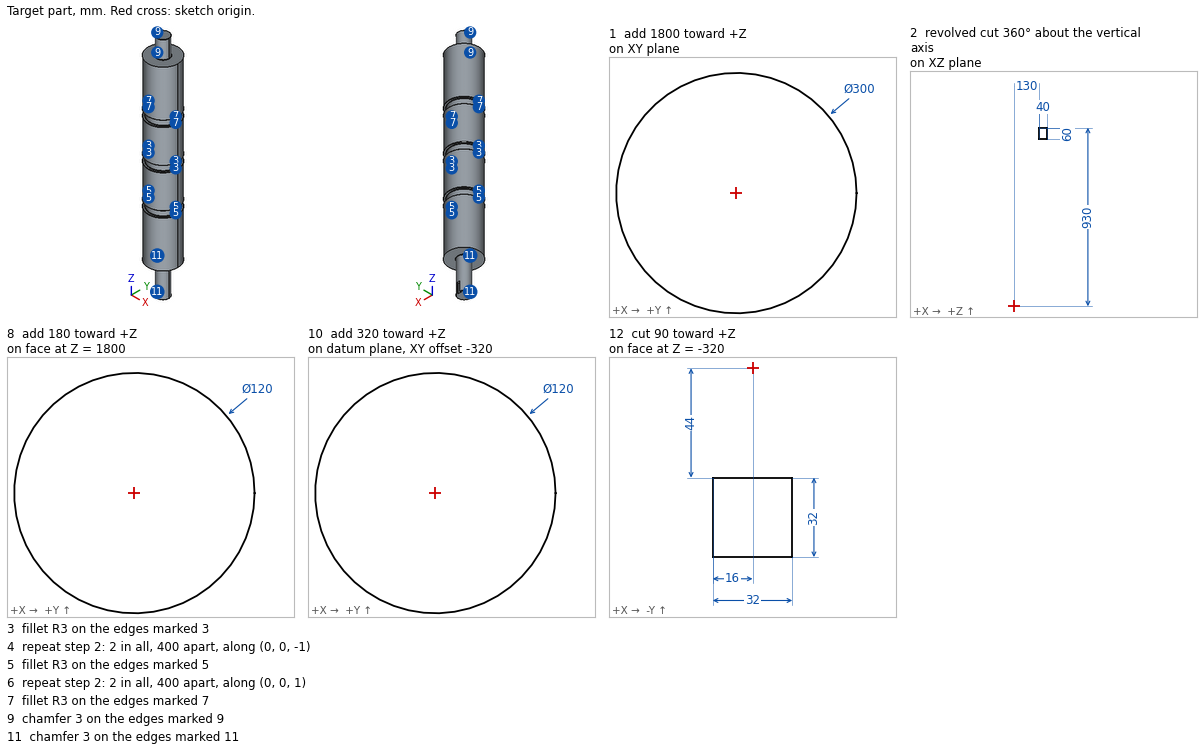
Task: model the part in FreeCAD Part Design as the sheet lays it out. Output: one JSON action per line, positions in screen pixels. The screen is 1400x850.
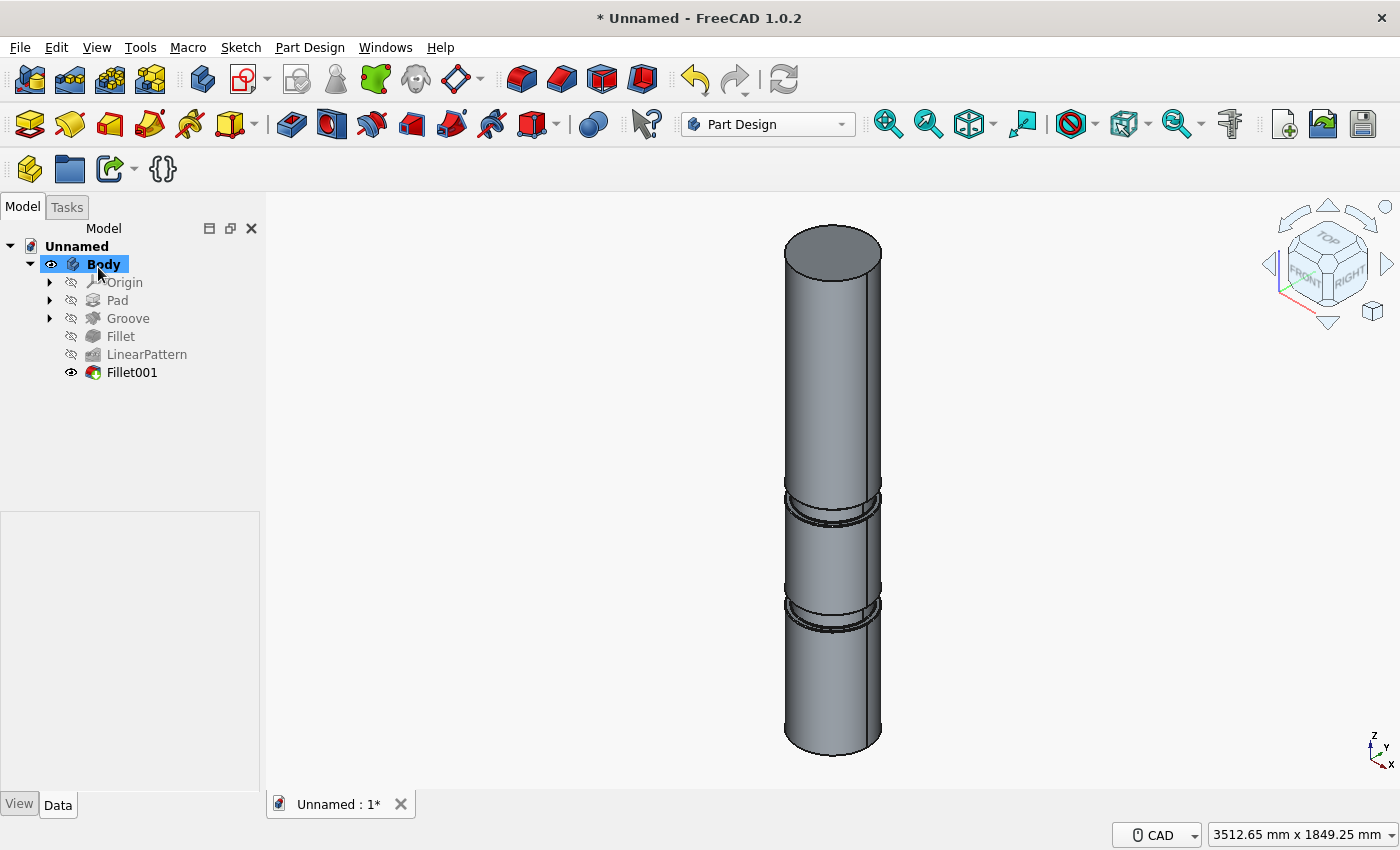
{"action": "left_click", "coordinate": [116, 318]}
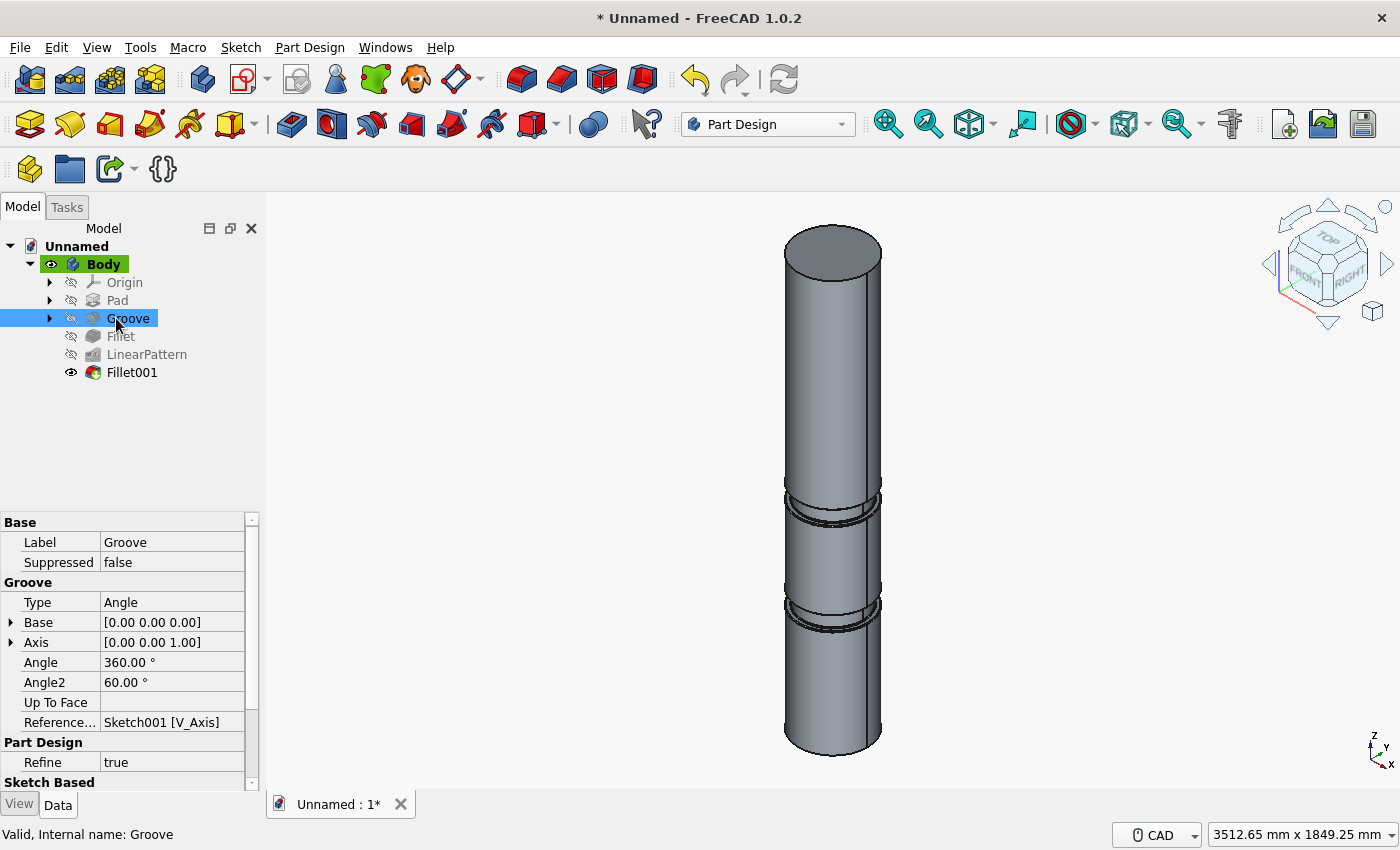
{"action": "left_click", "coordinate": [70, 80]}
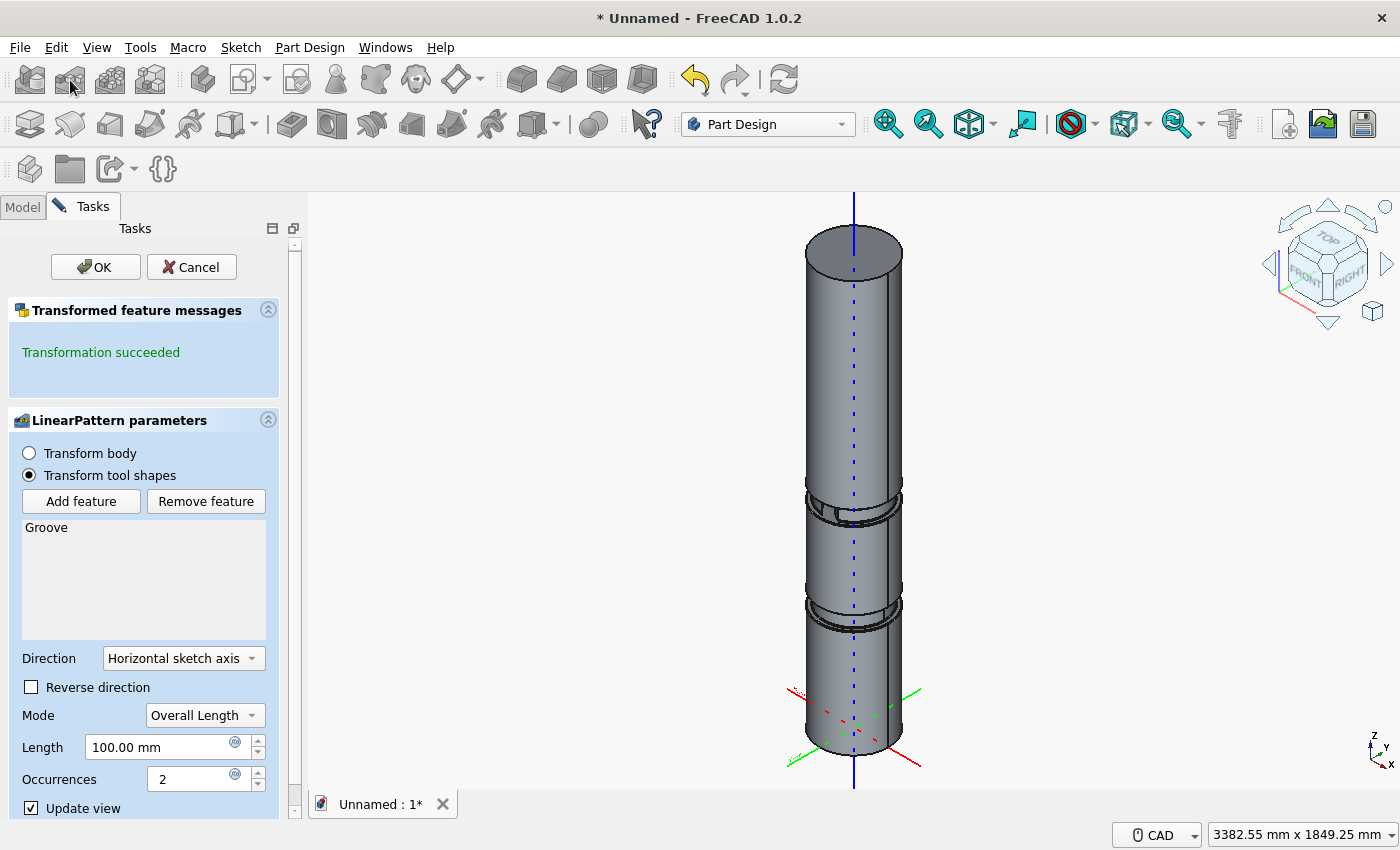
{"action": "left_click", "coordinate": [184, 658]}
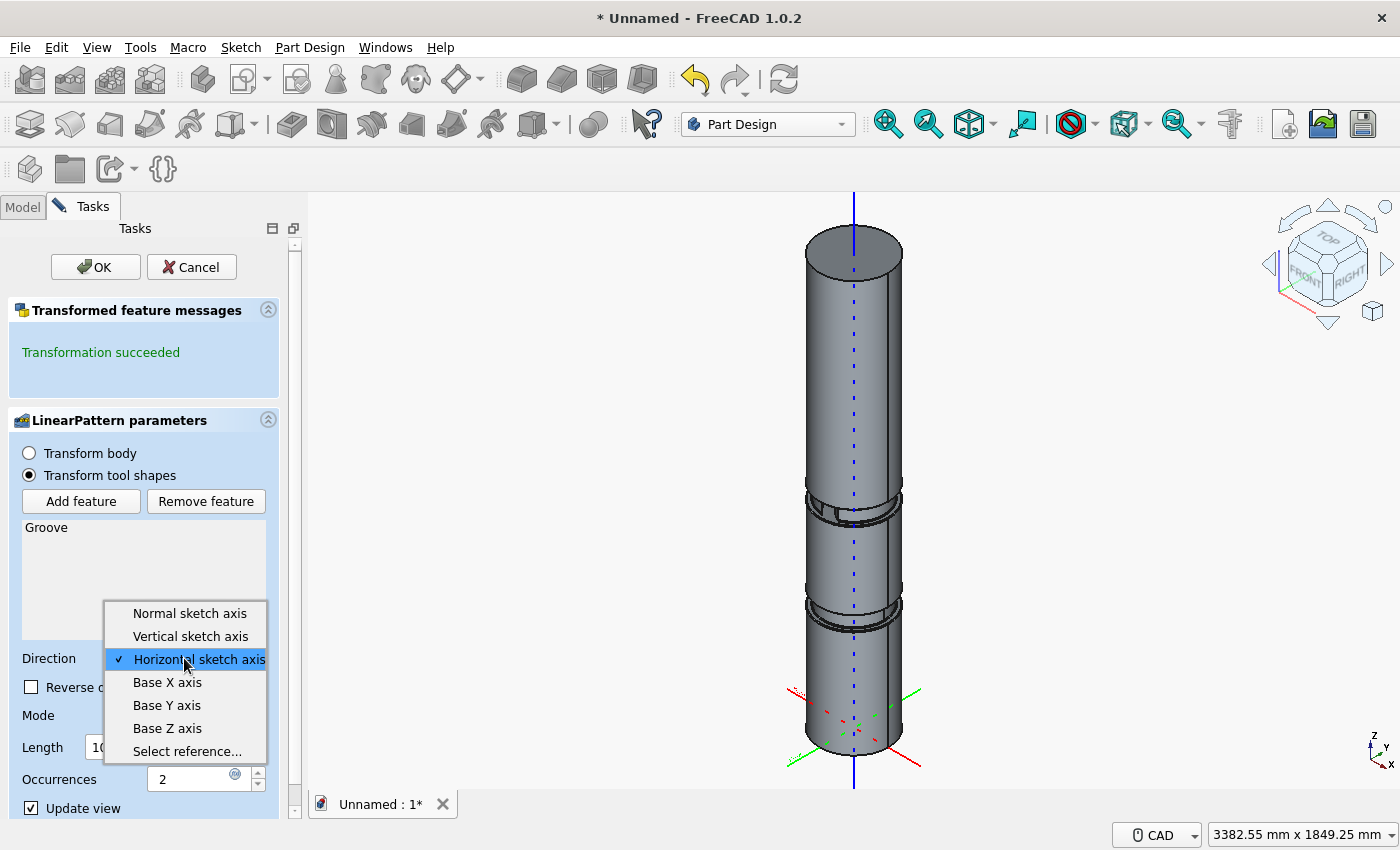
{"action": "left_click", "coordinate": [184, 728]}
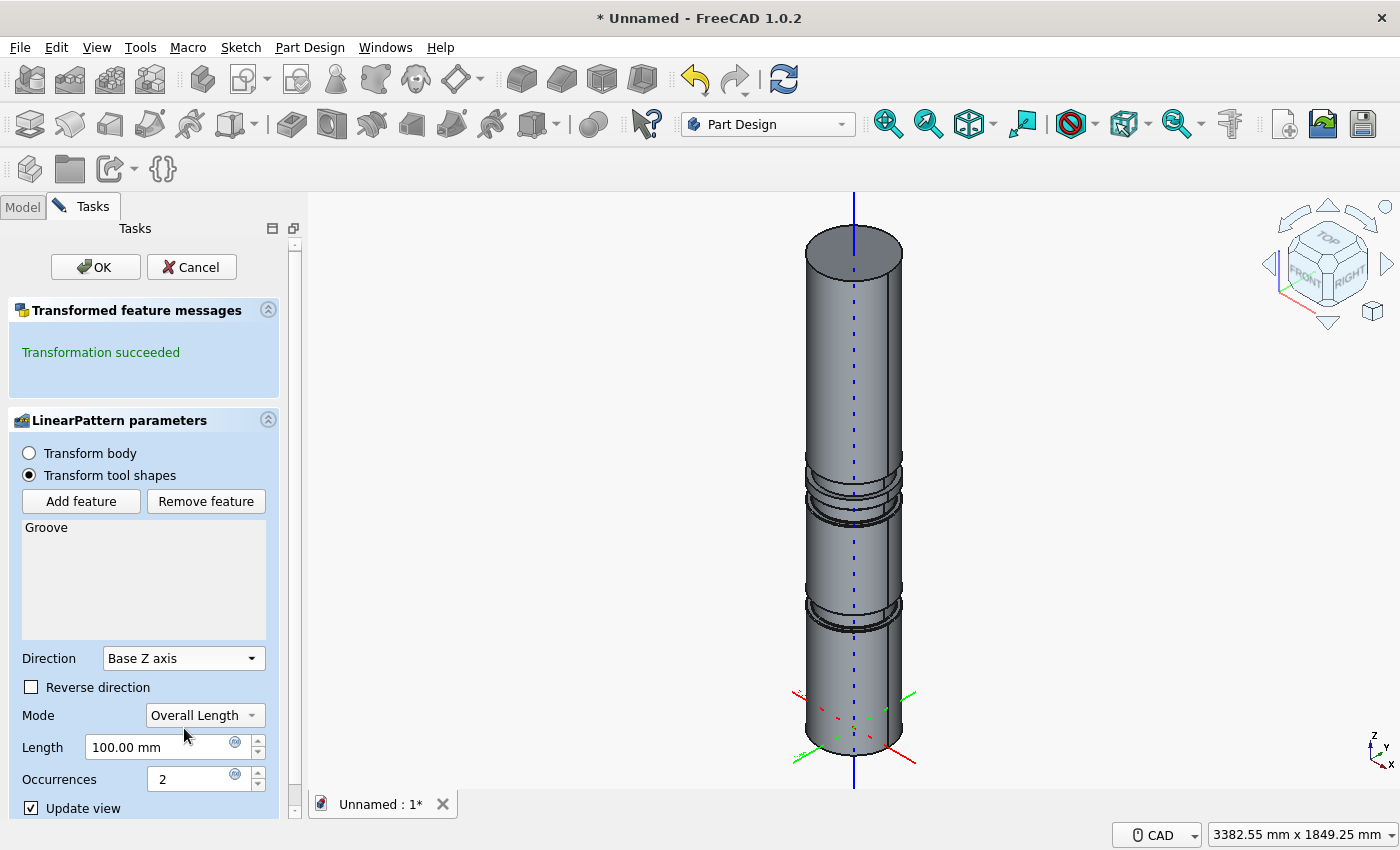
{"action": "left_click", "coordinate": [206, 716]}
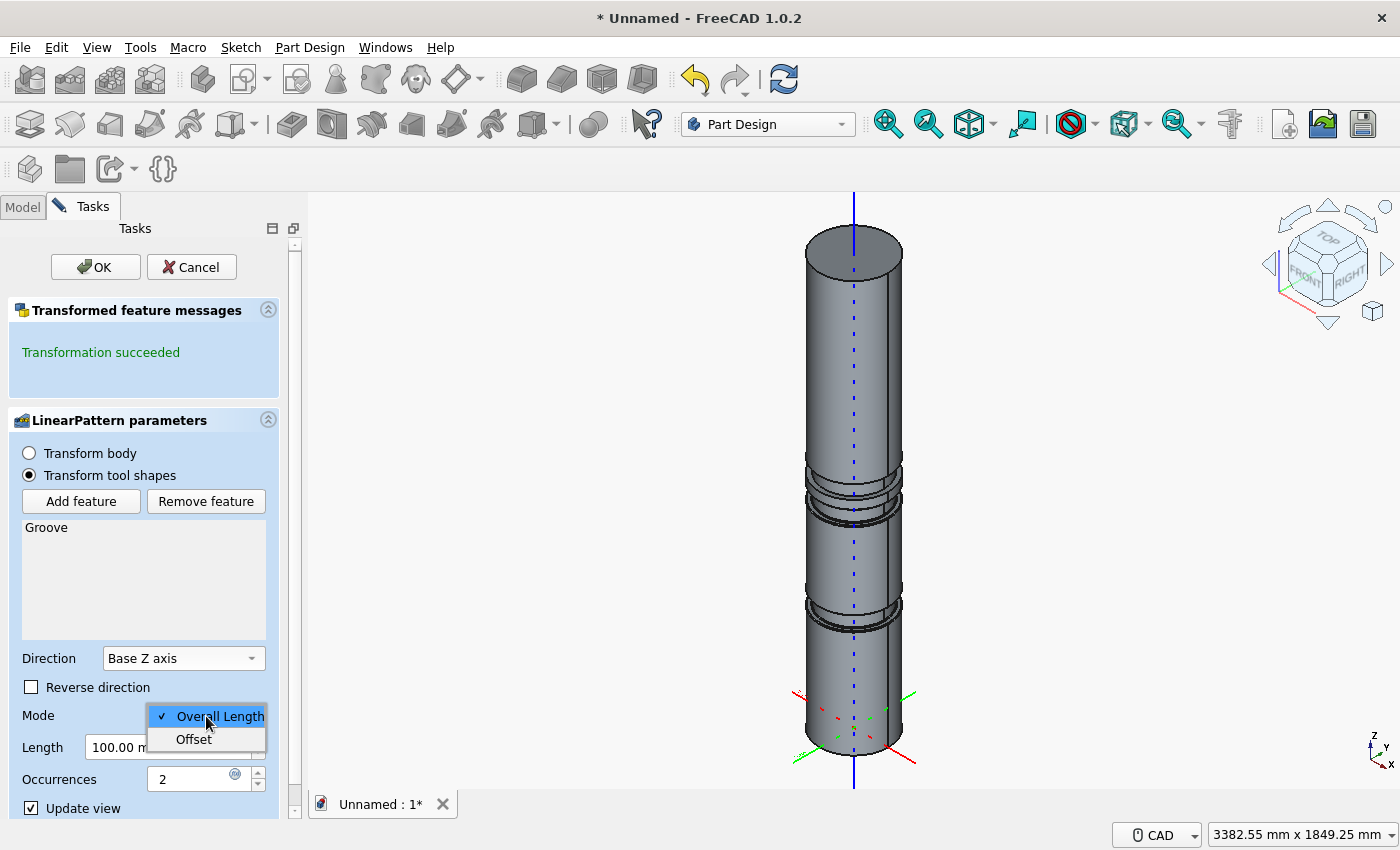
{"action": "left_click", "coordinate": [206, 740]}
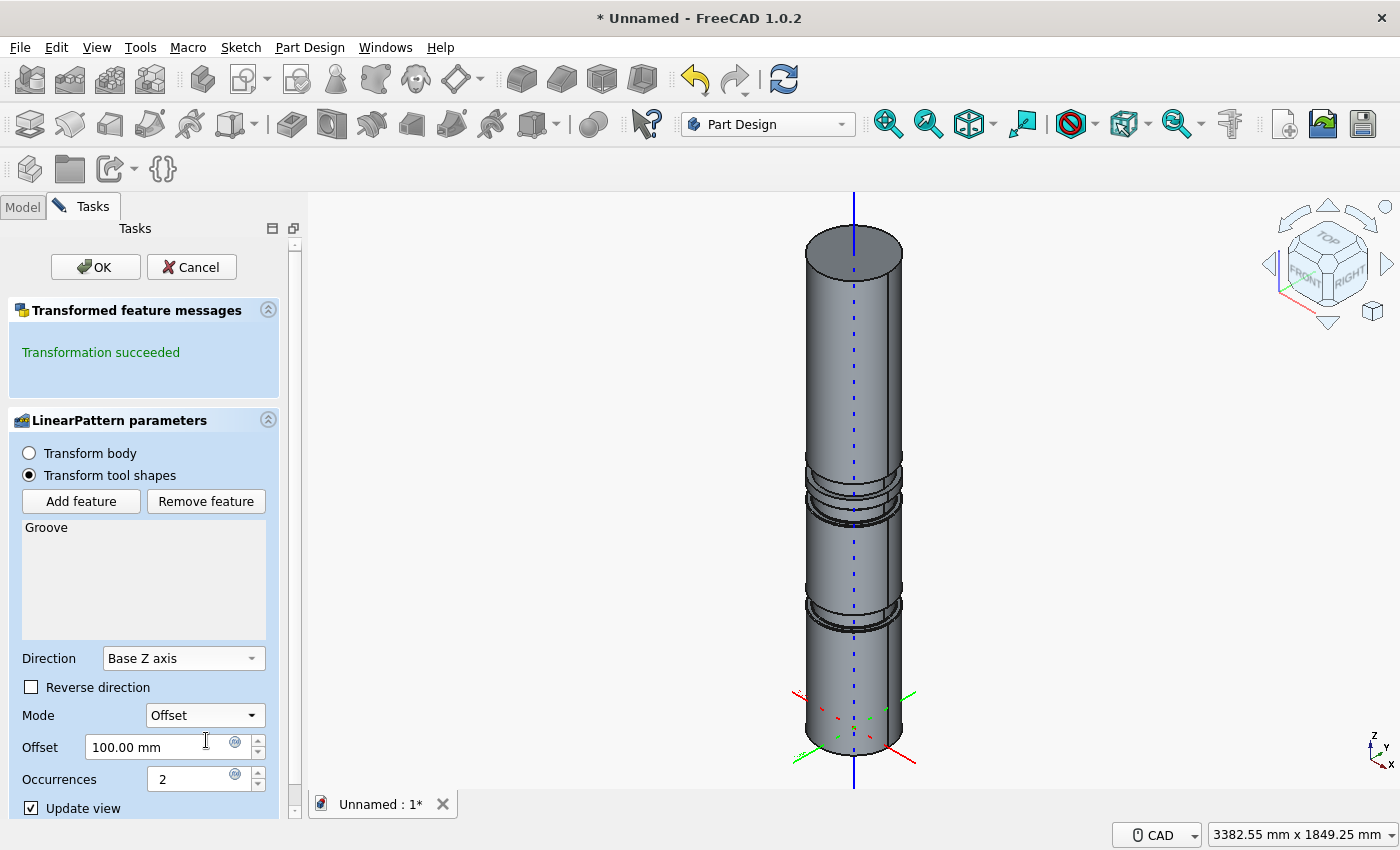
{"action": "triple_click", "coordinate": [168, 747]}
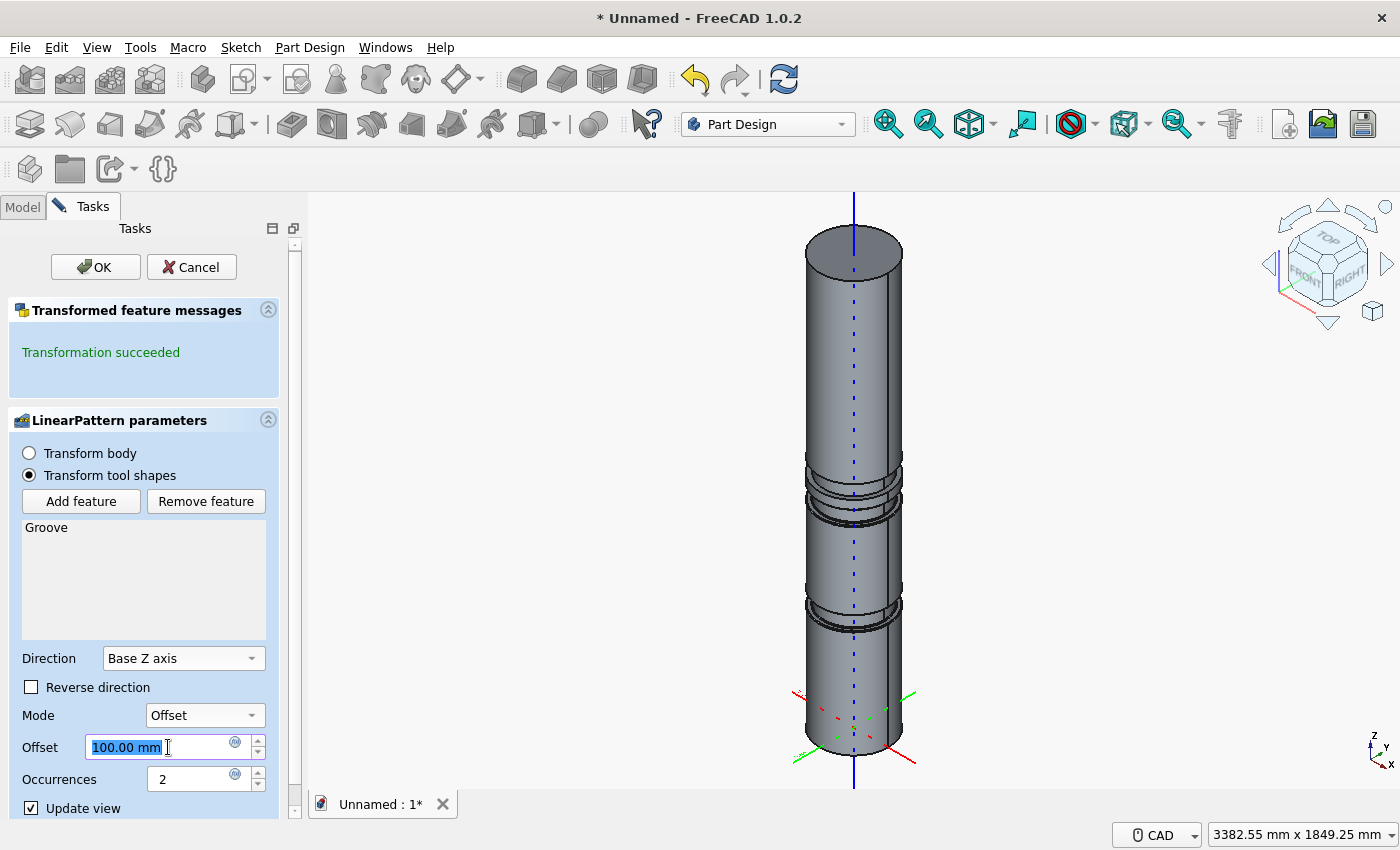
{"action": "type", "text": "400"}
{"action": "key", "text": "Tab"}